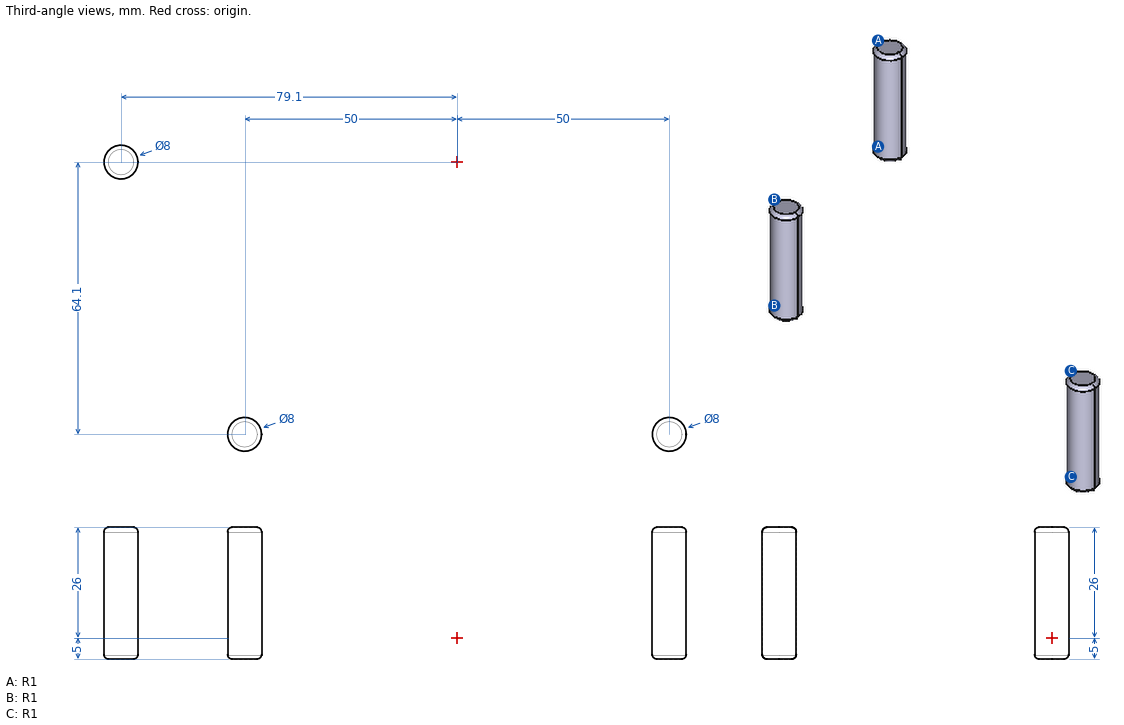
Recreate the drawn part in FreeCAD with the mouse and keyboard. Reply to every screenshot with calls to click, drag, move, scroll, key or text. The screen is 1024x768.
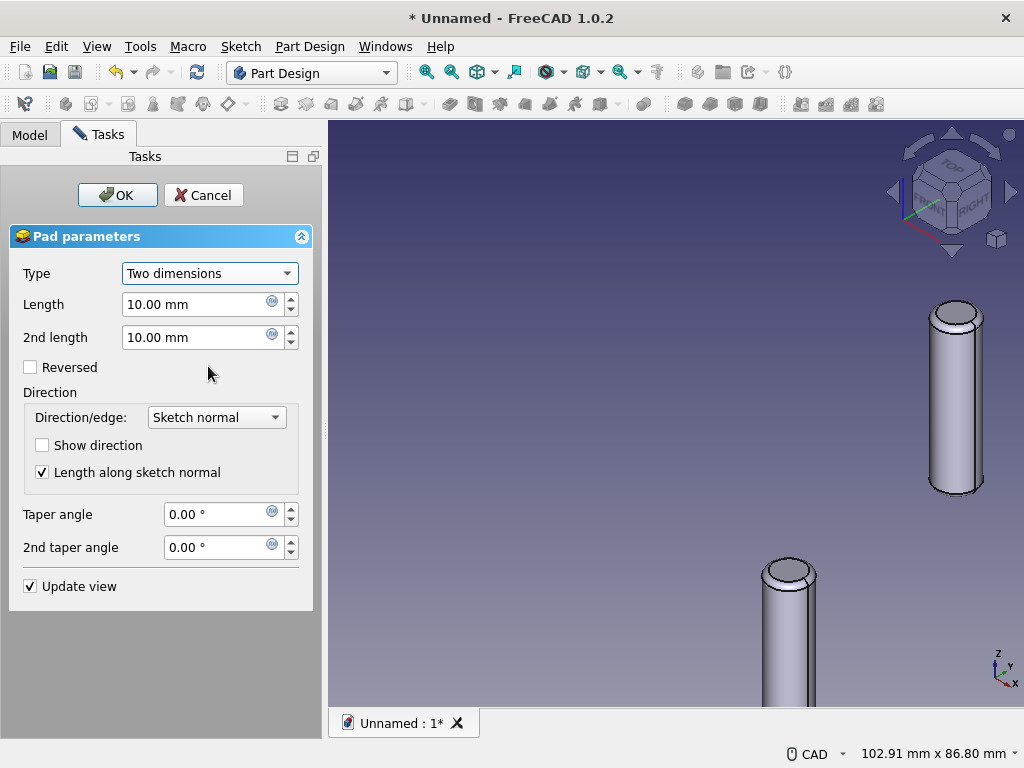
triple_click(204, 304)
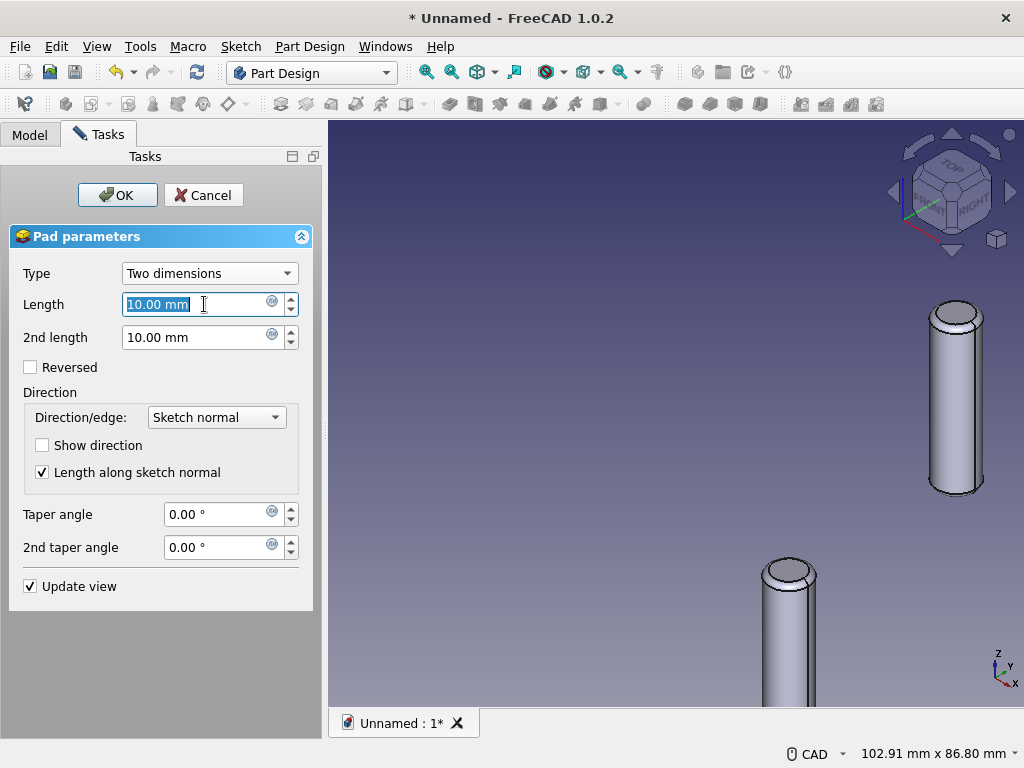
text(26)
key(Tab)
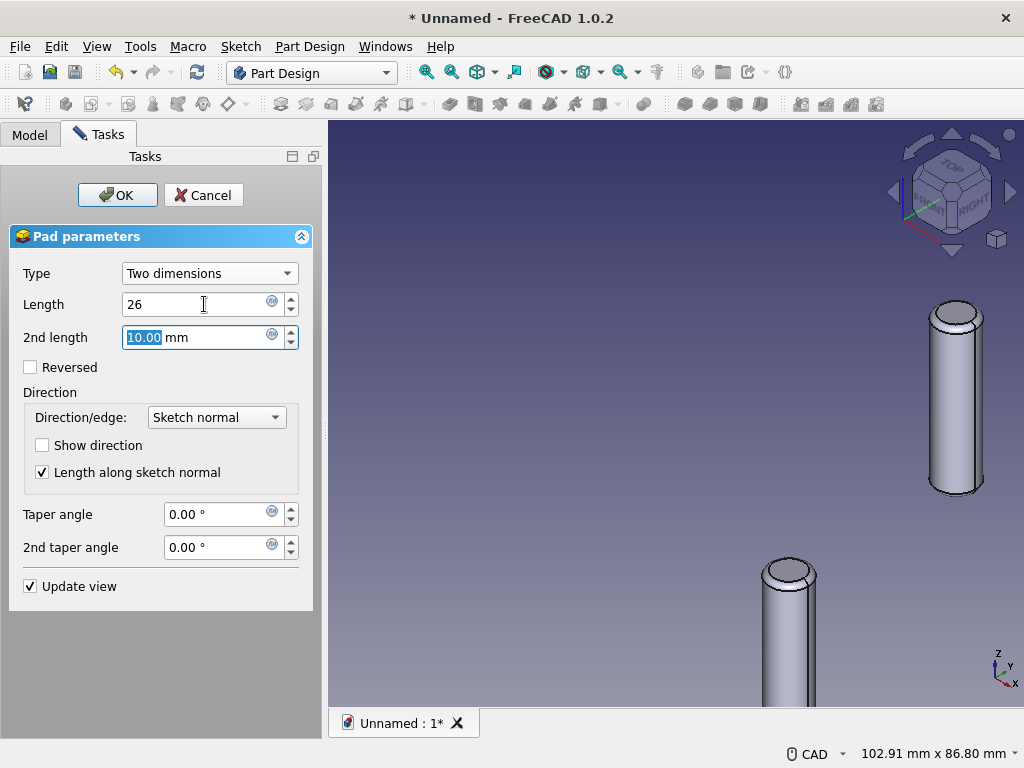
text(5)
key(Tab)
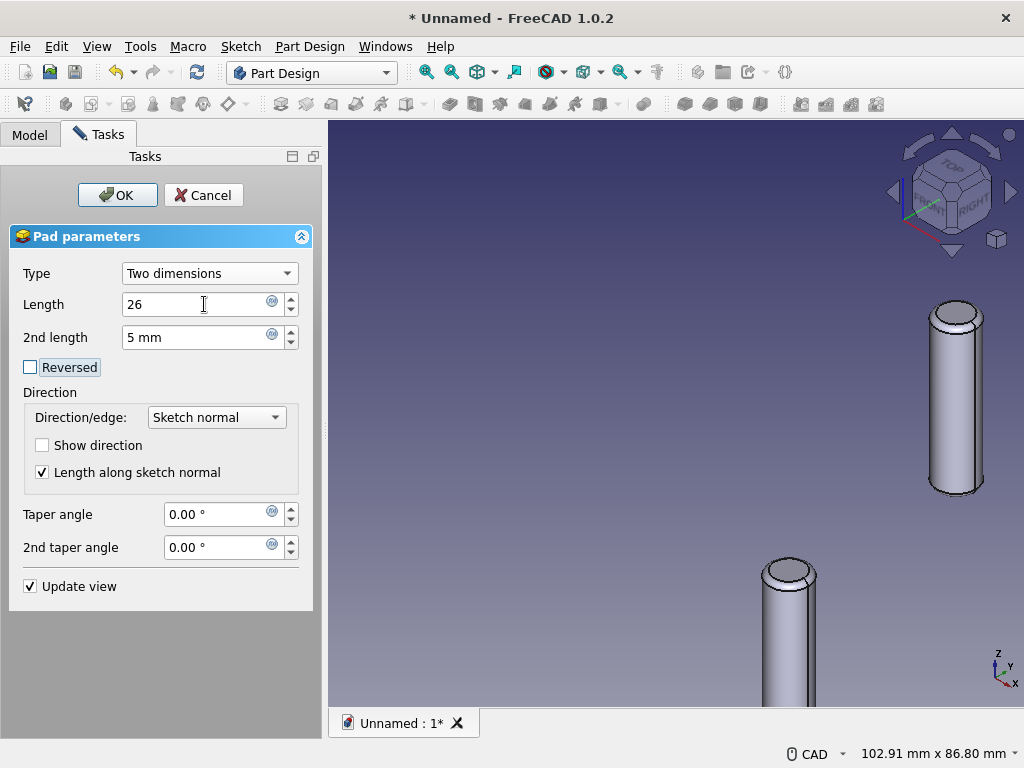
click(118, 195)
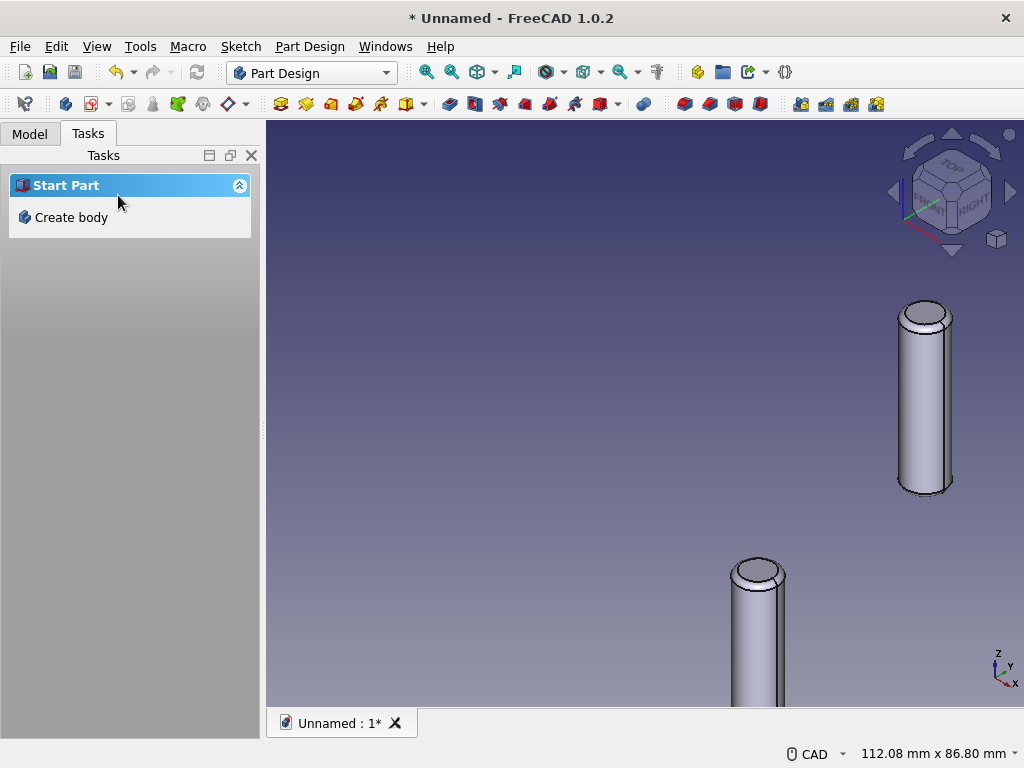
click(427, 72)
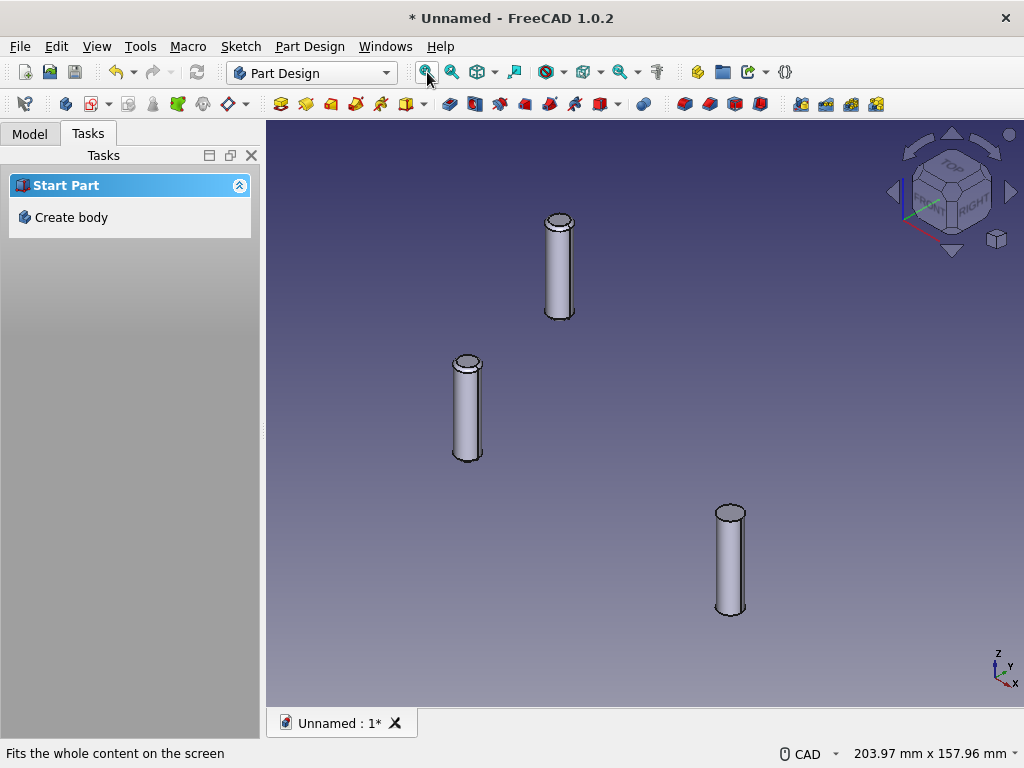
click(720, 506)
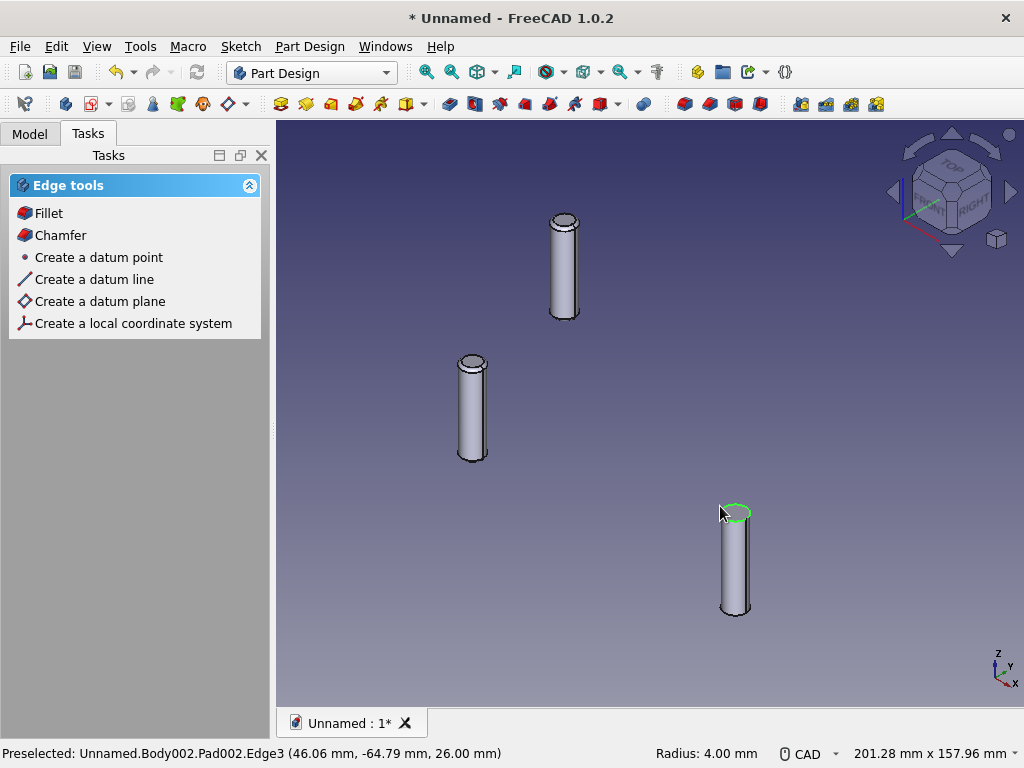
click(722, 610, ctrl)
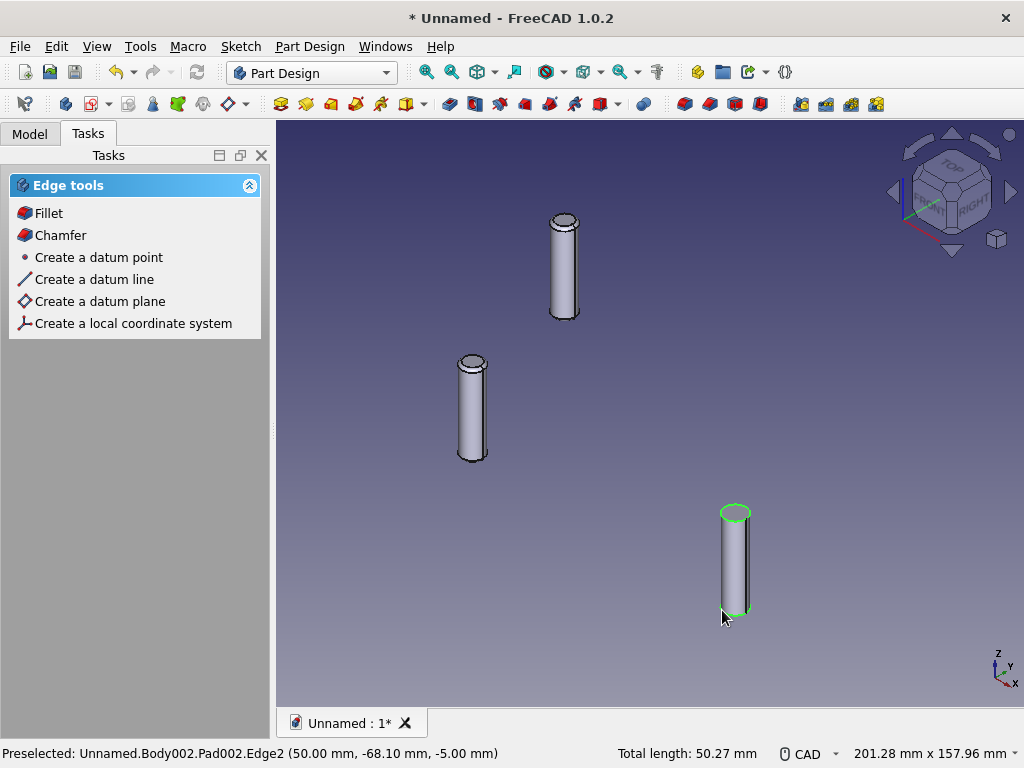
click(685, 104)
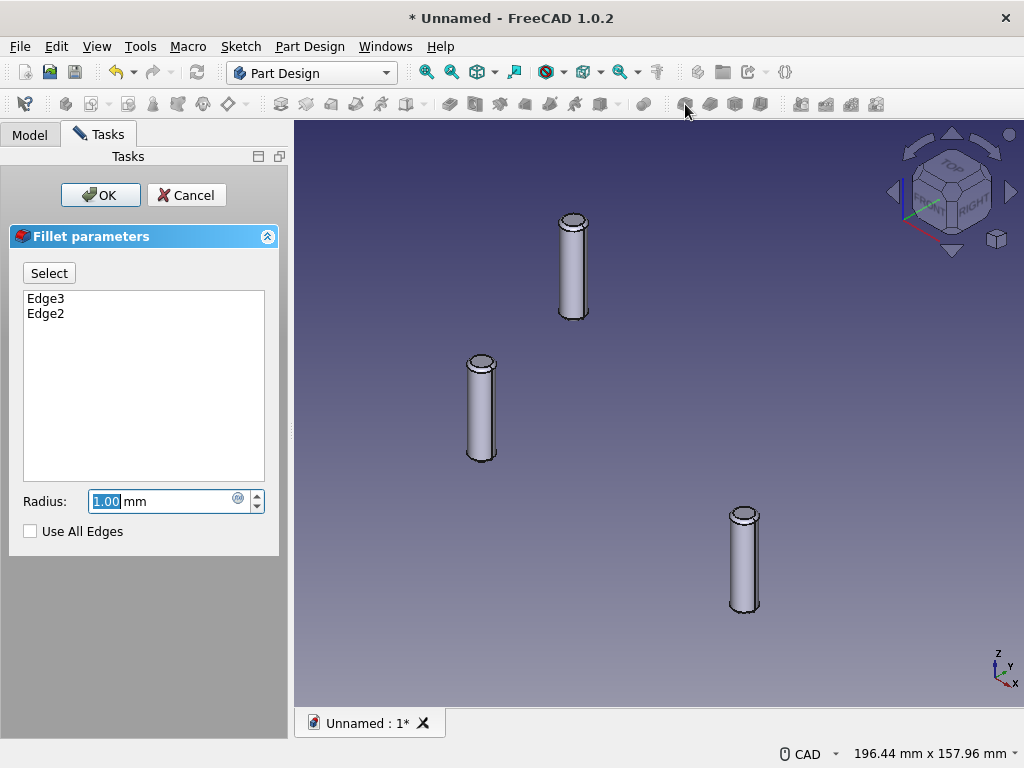
text(1)
key(Tab)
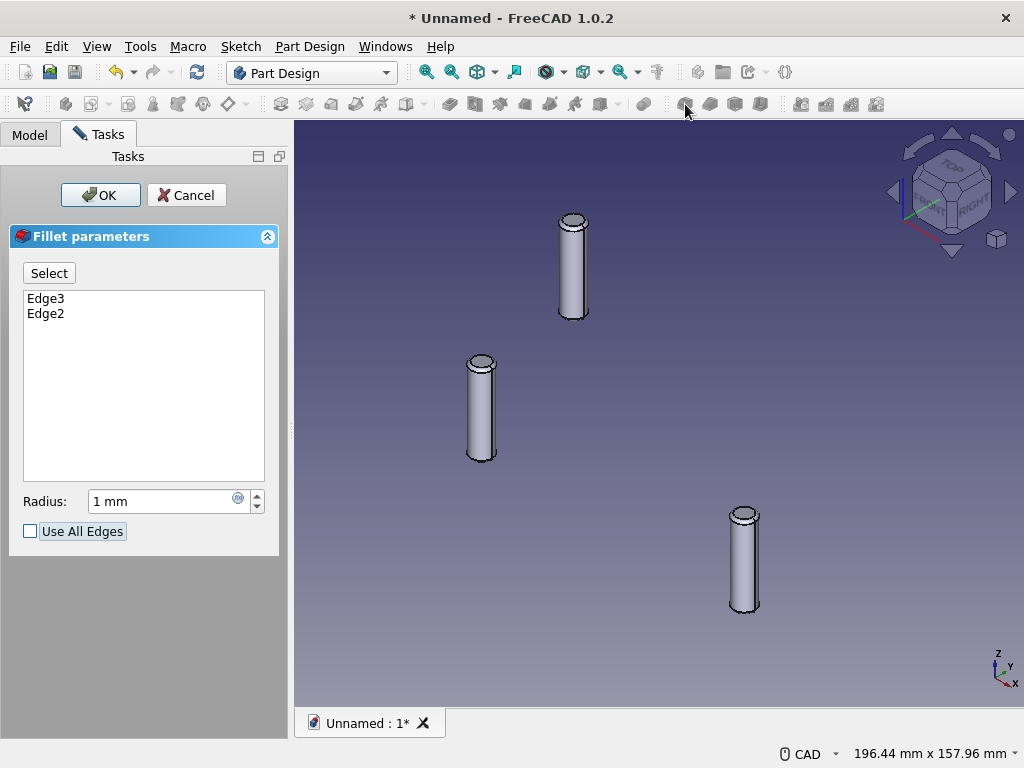
click(101, 195)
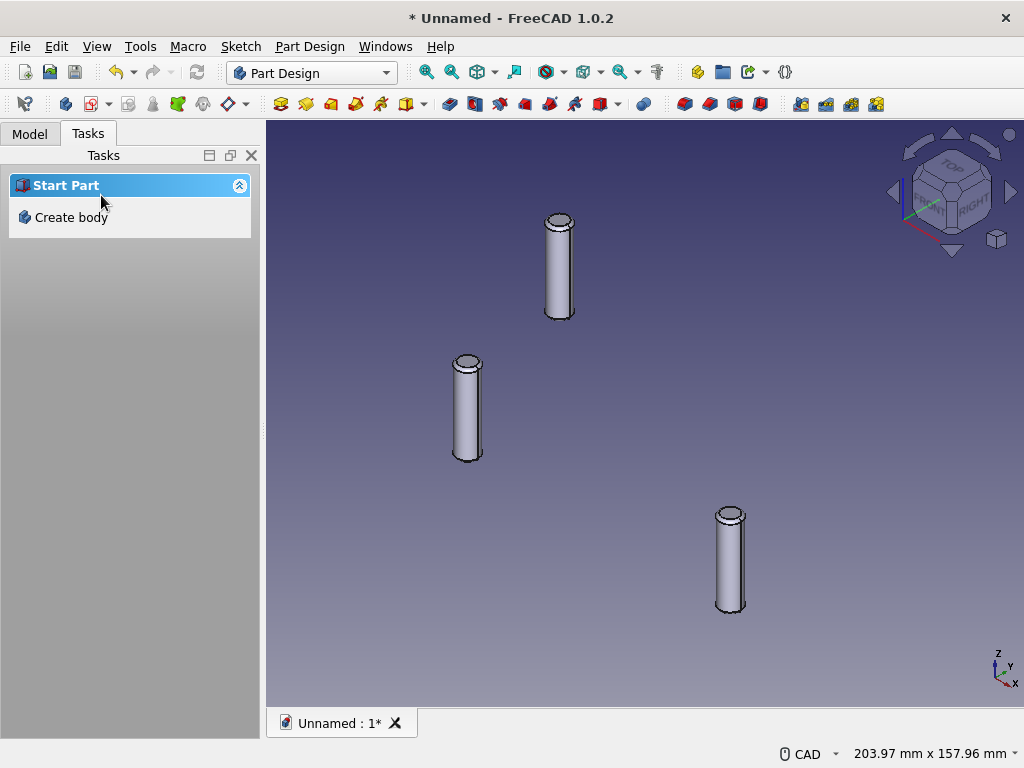
click(427, 72)